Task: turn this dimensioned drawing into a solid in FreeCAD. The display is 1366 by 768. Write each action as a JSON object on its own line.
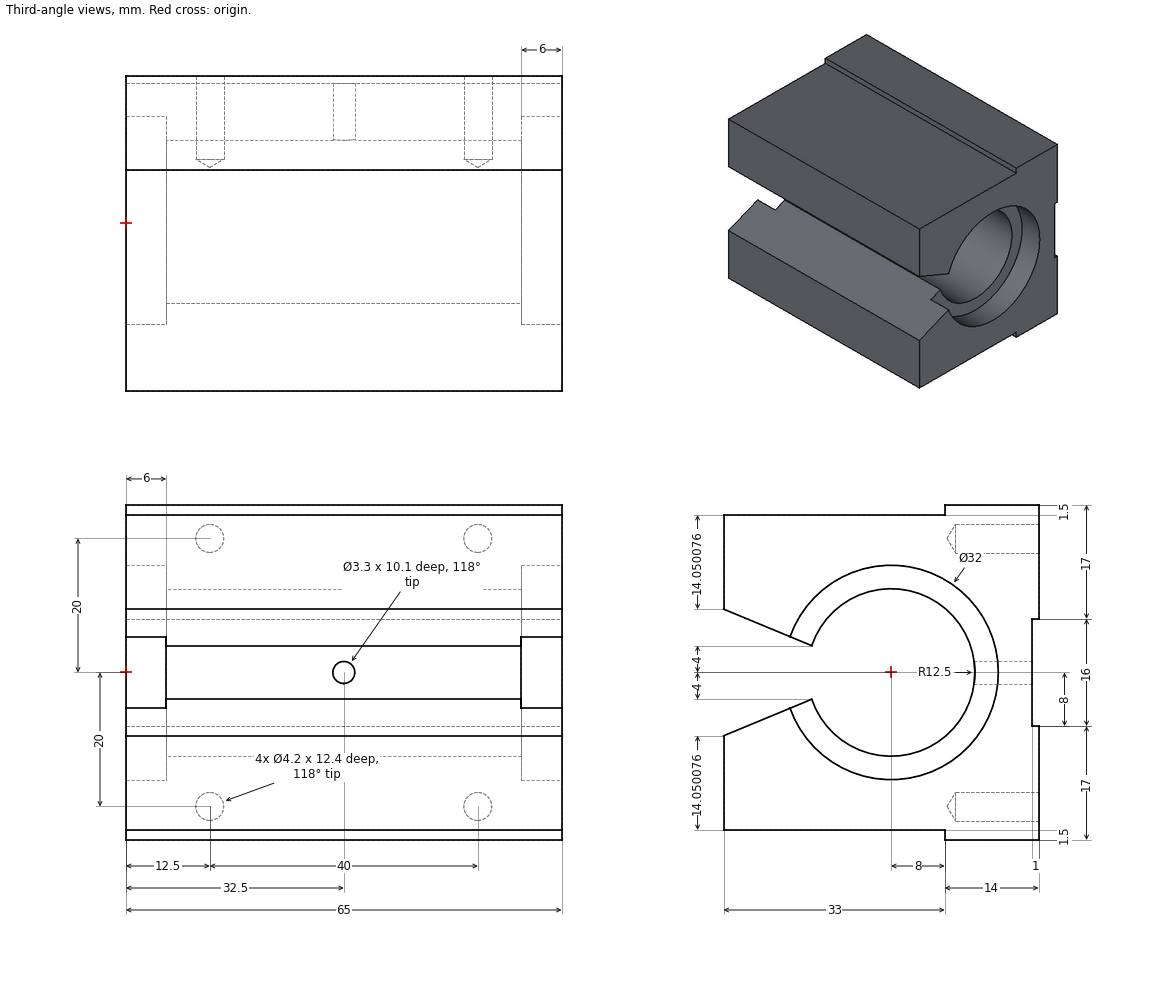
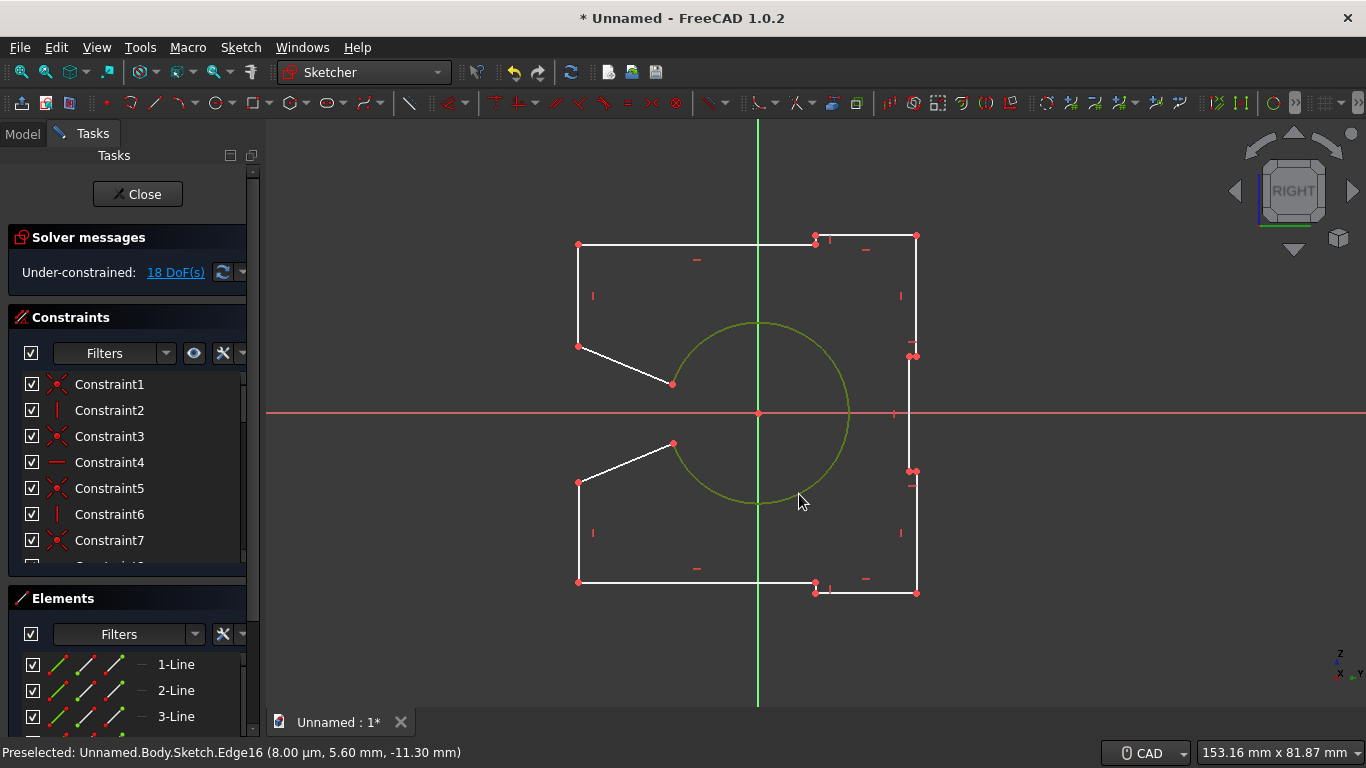
{"action": "key", "text": "k r"}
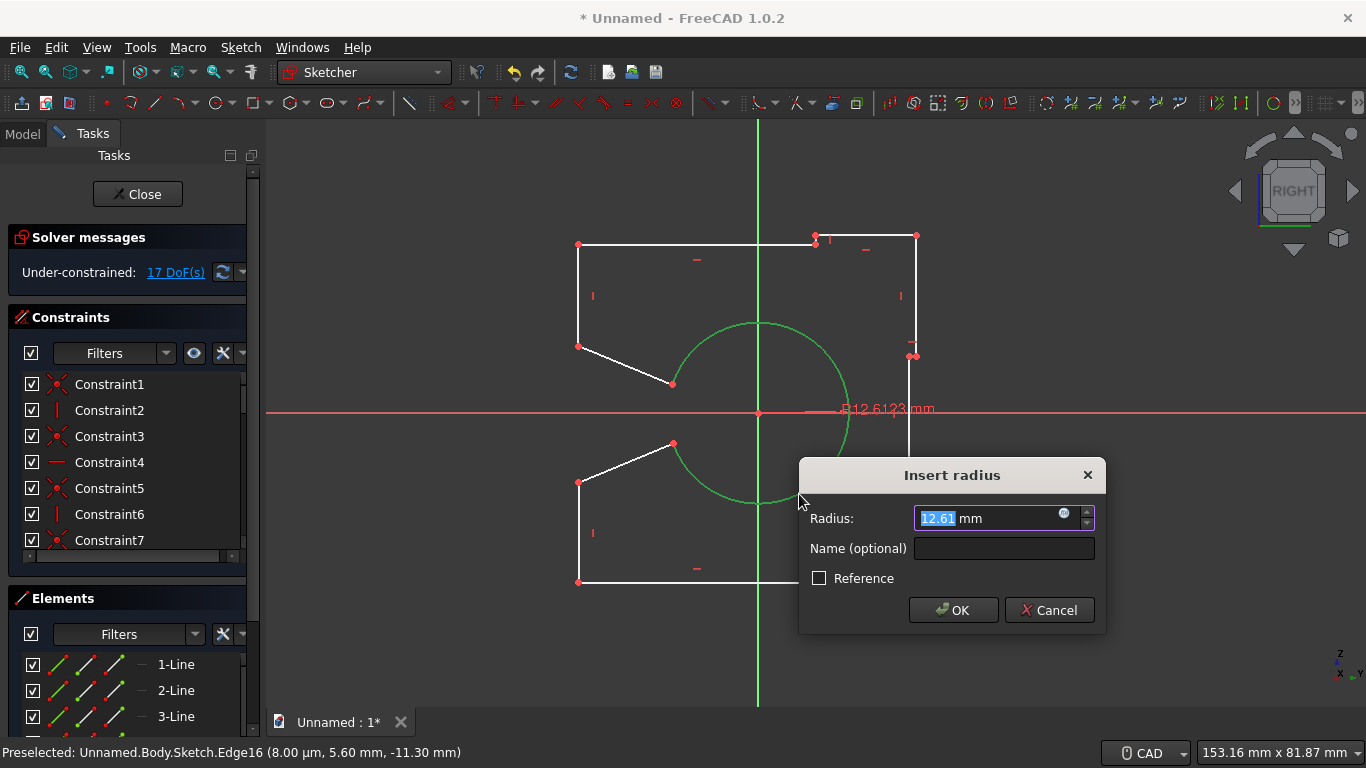
{"action": "type", "text": "12.5"}
{"action": "key", "text": "Return"}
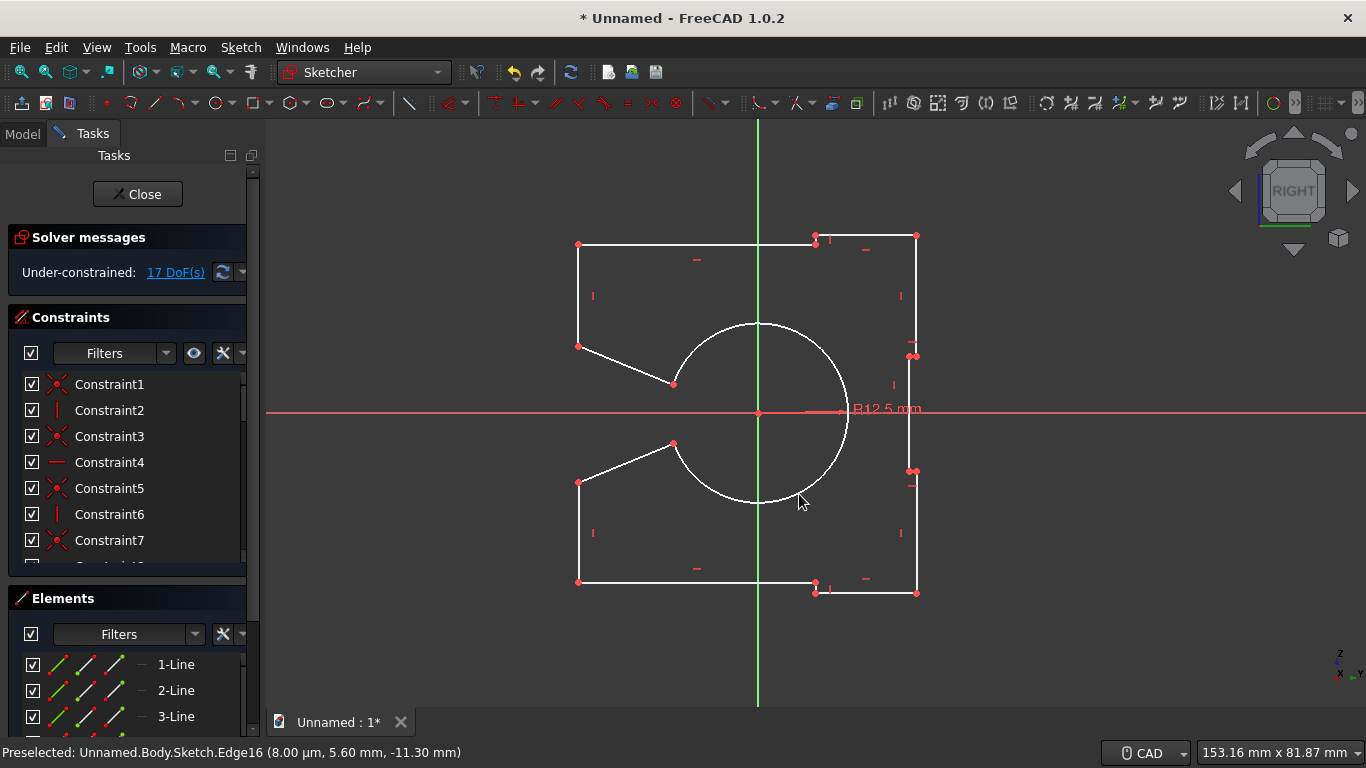
{"action": "scroll", "coordinate": [913, 471], "scroll_direction": "up", "scroll_amount": 9}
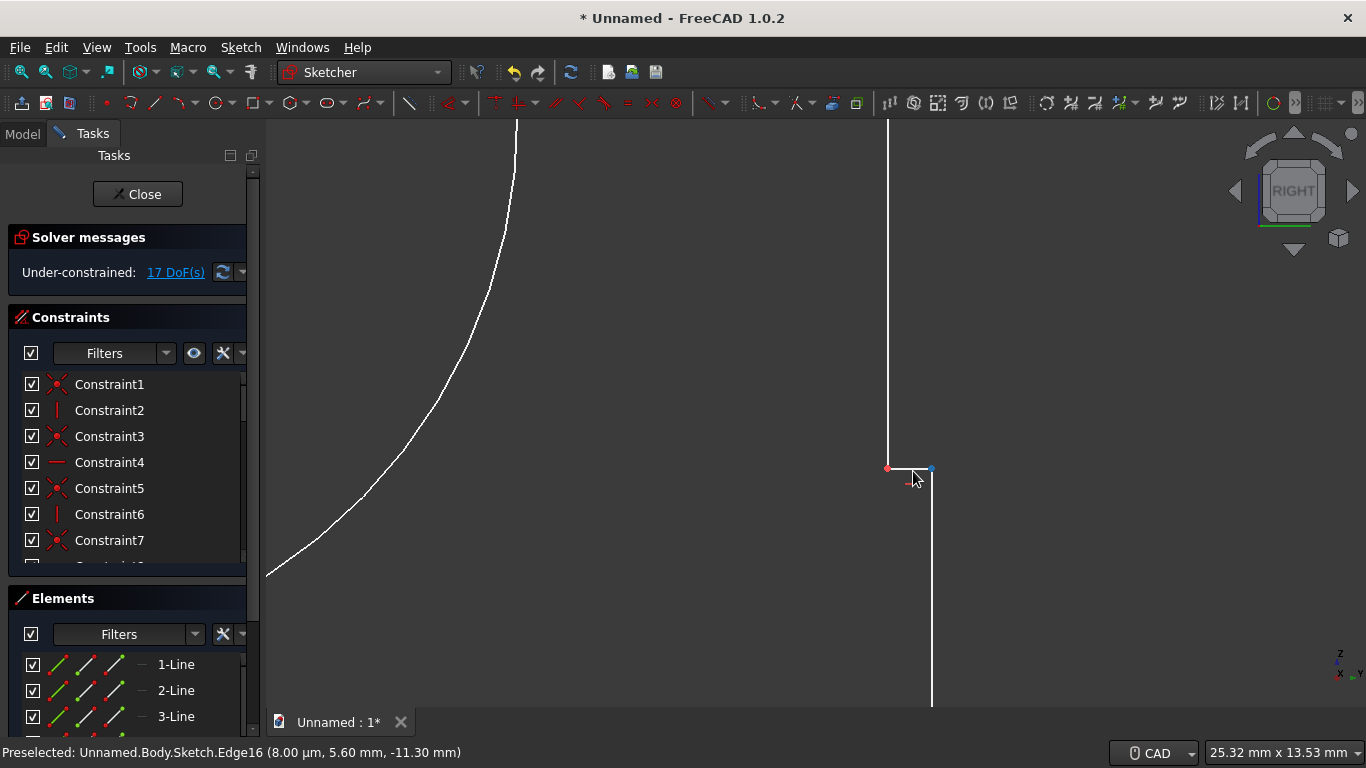
{"action": "left_click", "coordinate": [910, 469]}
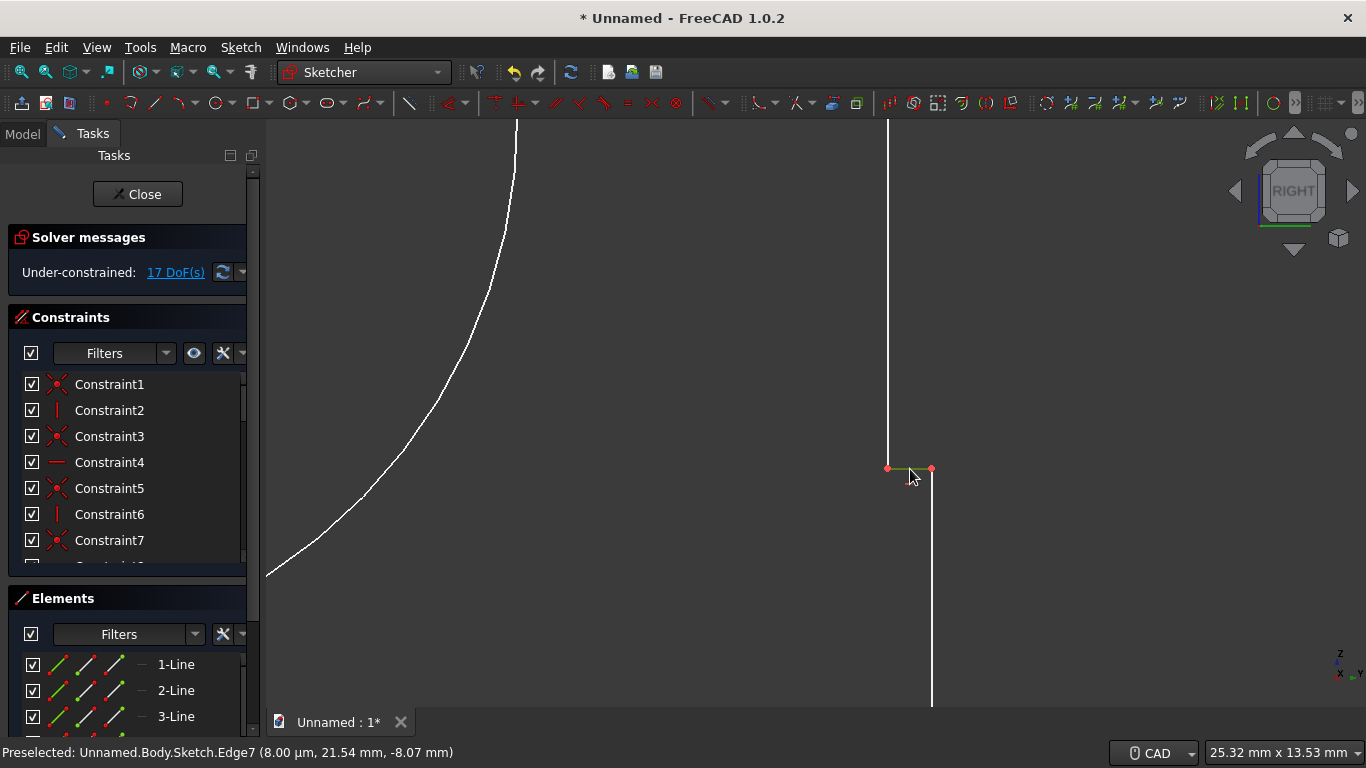
{"action": "key", "text": "l"}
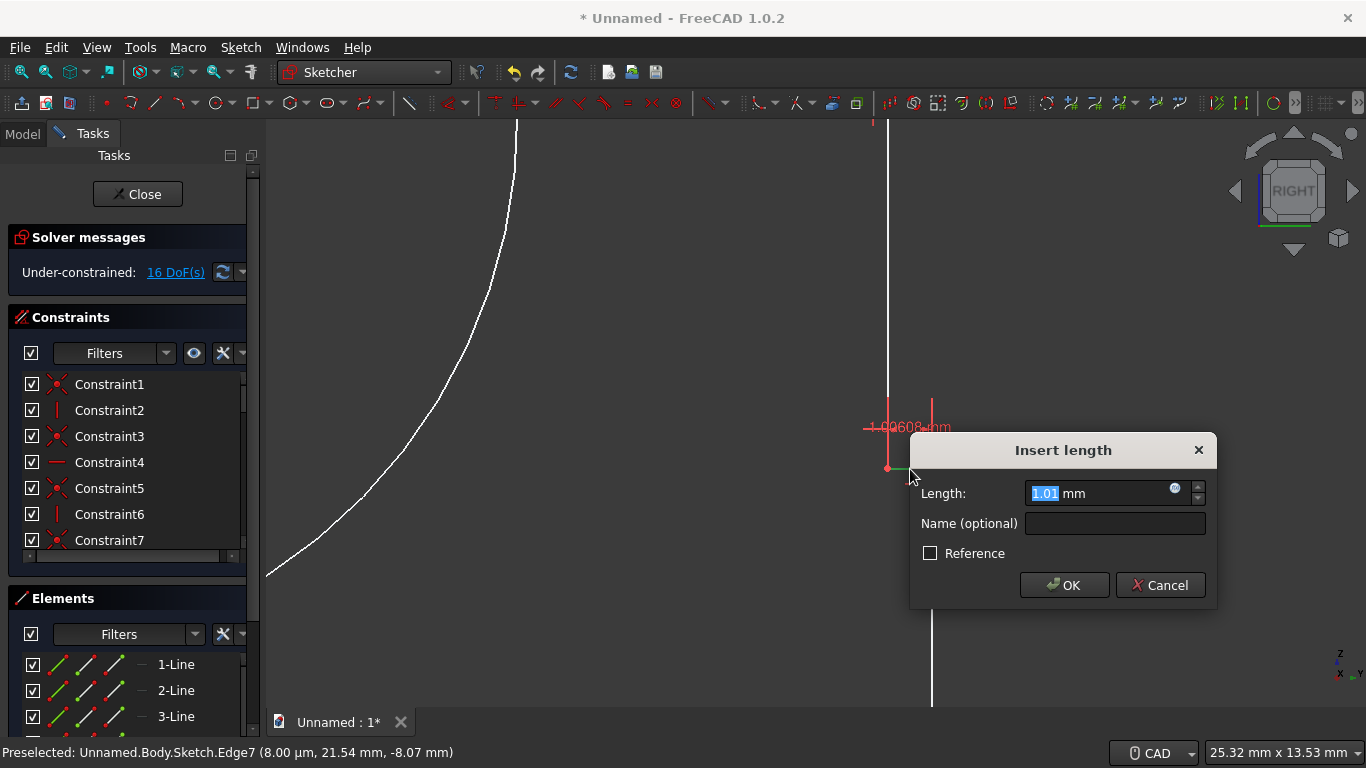
{"action": "type", "text": "1"}
{"action": "key", "text": "Return"}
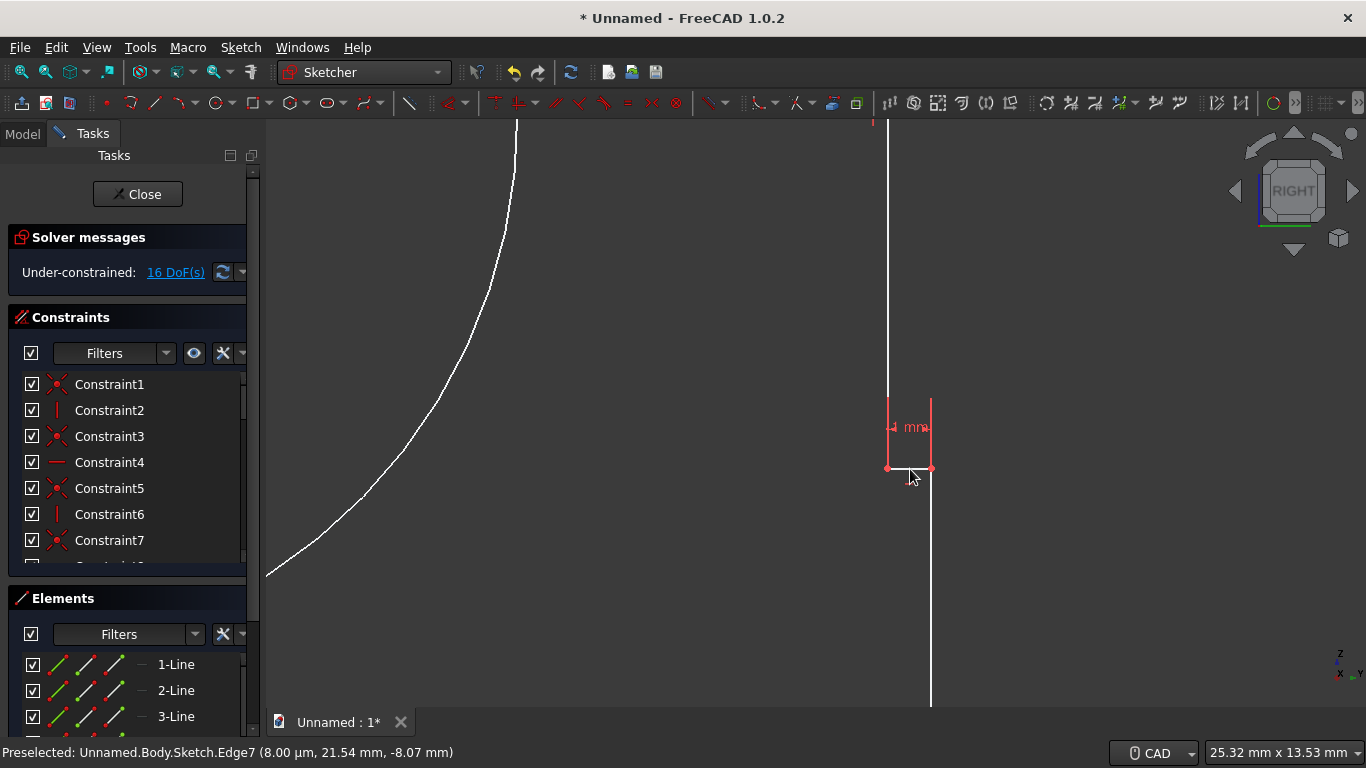
{"action": "scroll", "coordinate": [914, 471], "scroll_direction": "down", "scroll_amount": 9}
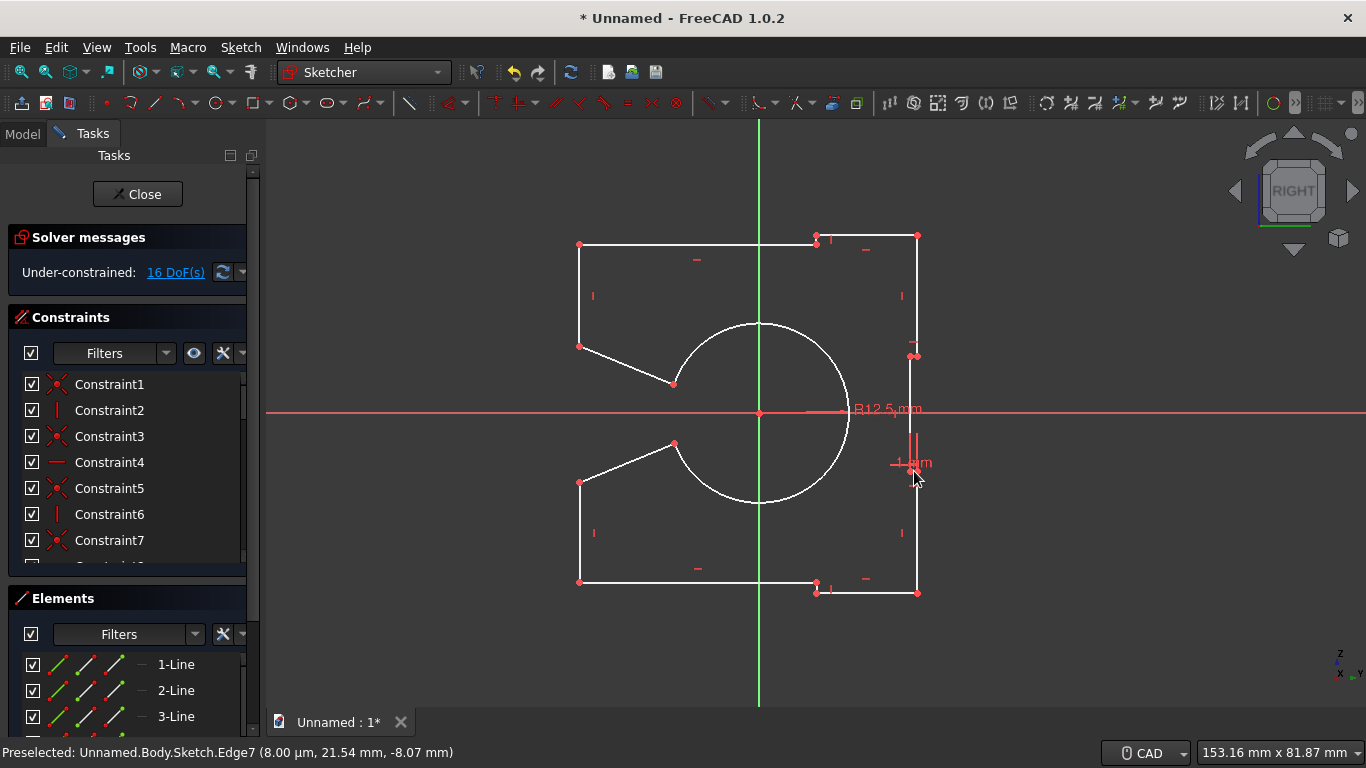
{"action": "scroll", "coordinate": [912, 357], "scroll_direction": "up", "scroll_amount": 10}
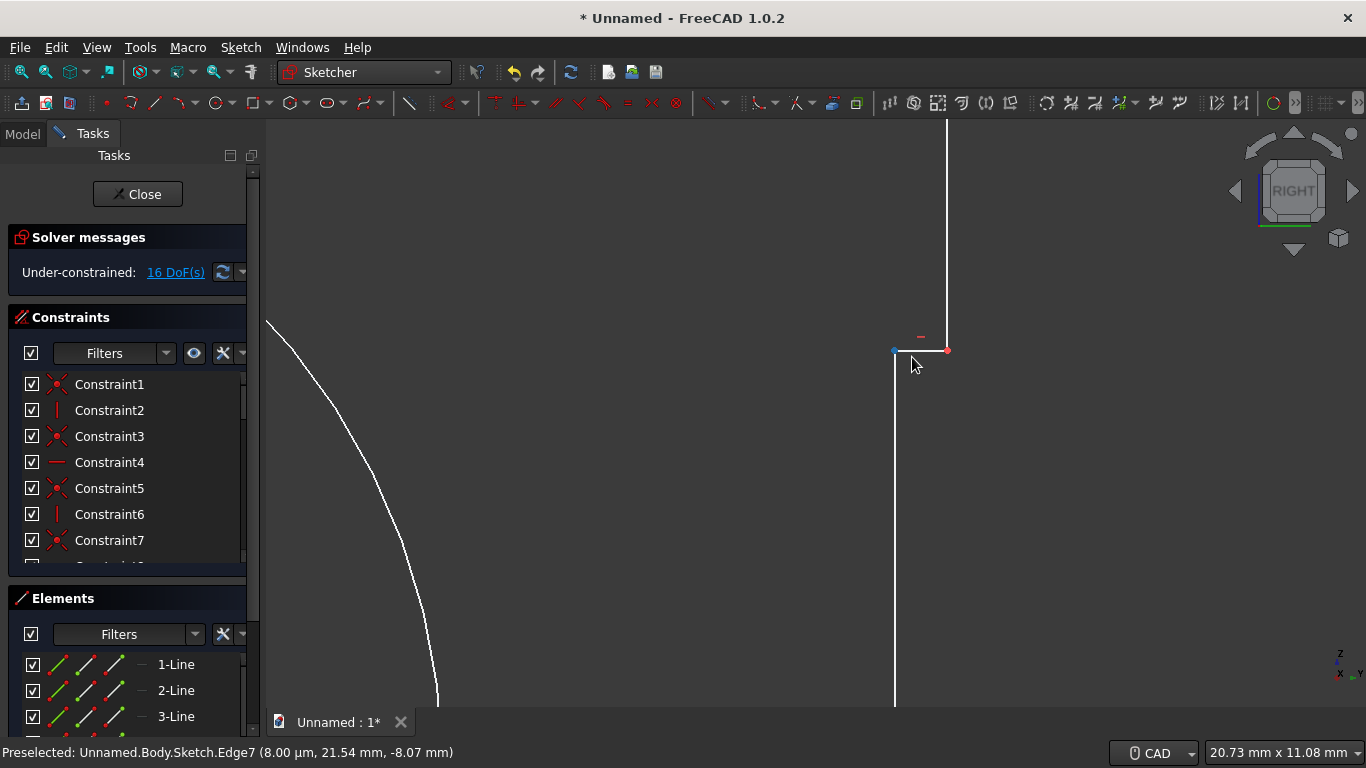
{"action": "left_click", "coordinate": [911, 351]}